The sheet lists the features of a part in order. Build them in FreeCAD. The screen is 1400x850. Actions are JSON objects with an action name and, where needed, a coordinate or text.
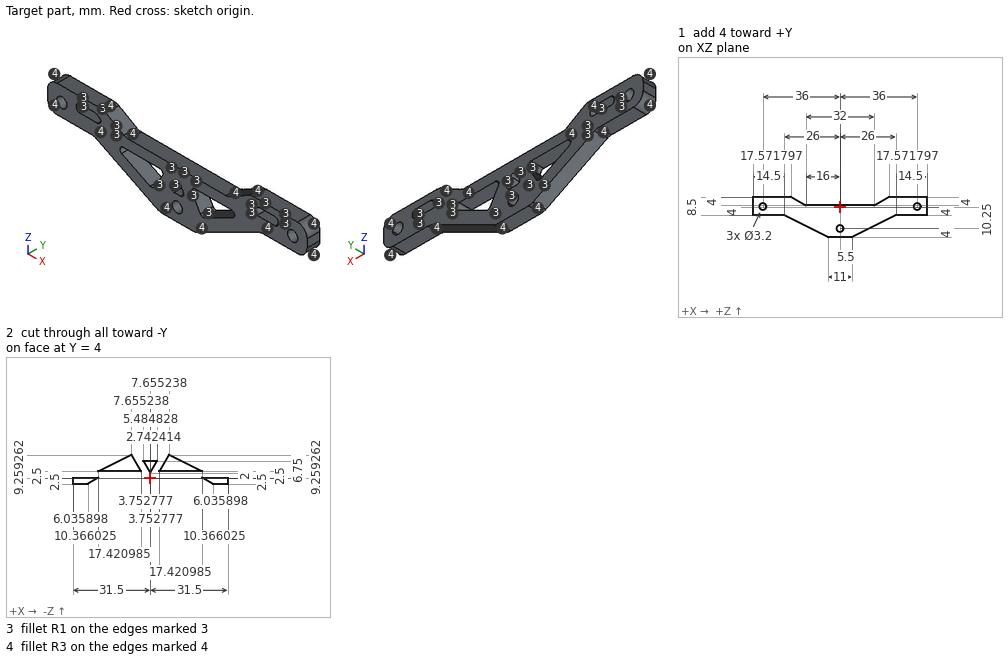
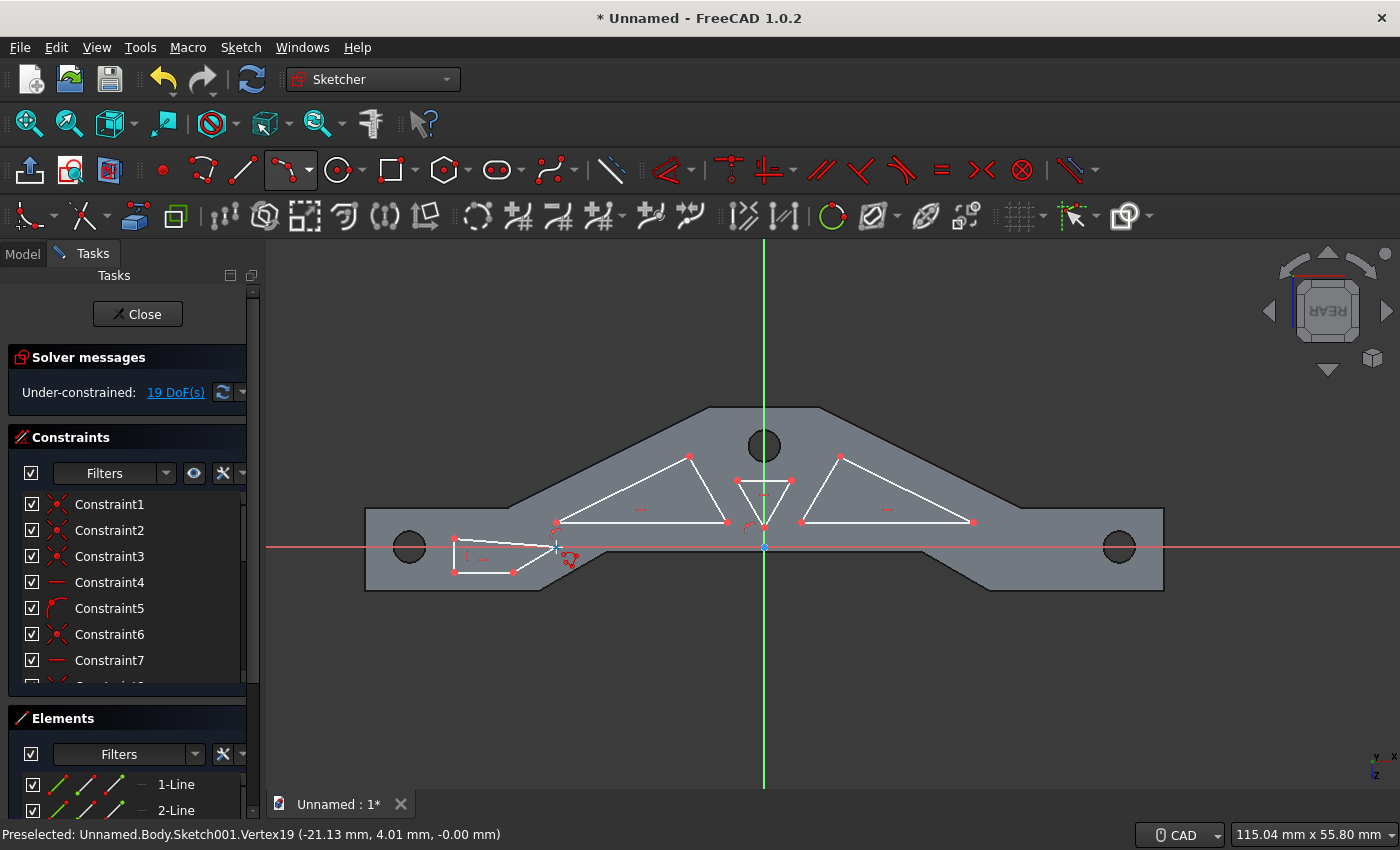
{"action": "left_click", "coordinate": [973, 547]}
{"action": "left_click", "coordinate": [1015, 572]}
{"action": "left_click", "coordinate": [1075, 572]}
{"action": "left_click", "coordinate": [1075, 538]}
{"action": "left_click", "coordinate": [973, 547]}
{"action": "key", "text": "Escape"}
{"action": "key", "text": "Escape"}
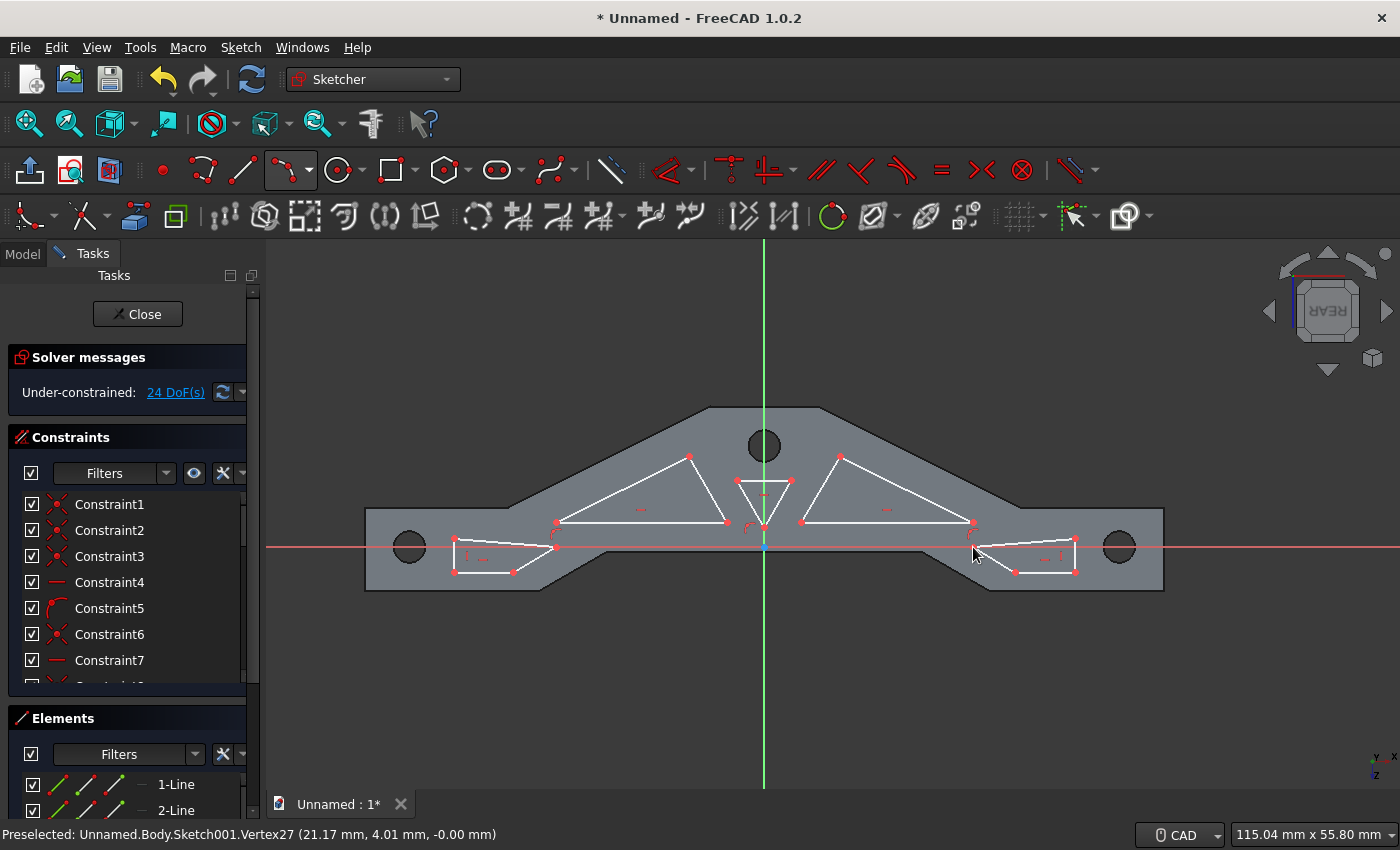
{"action": "left_click", "coordinate": [525, 545]}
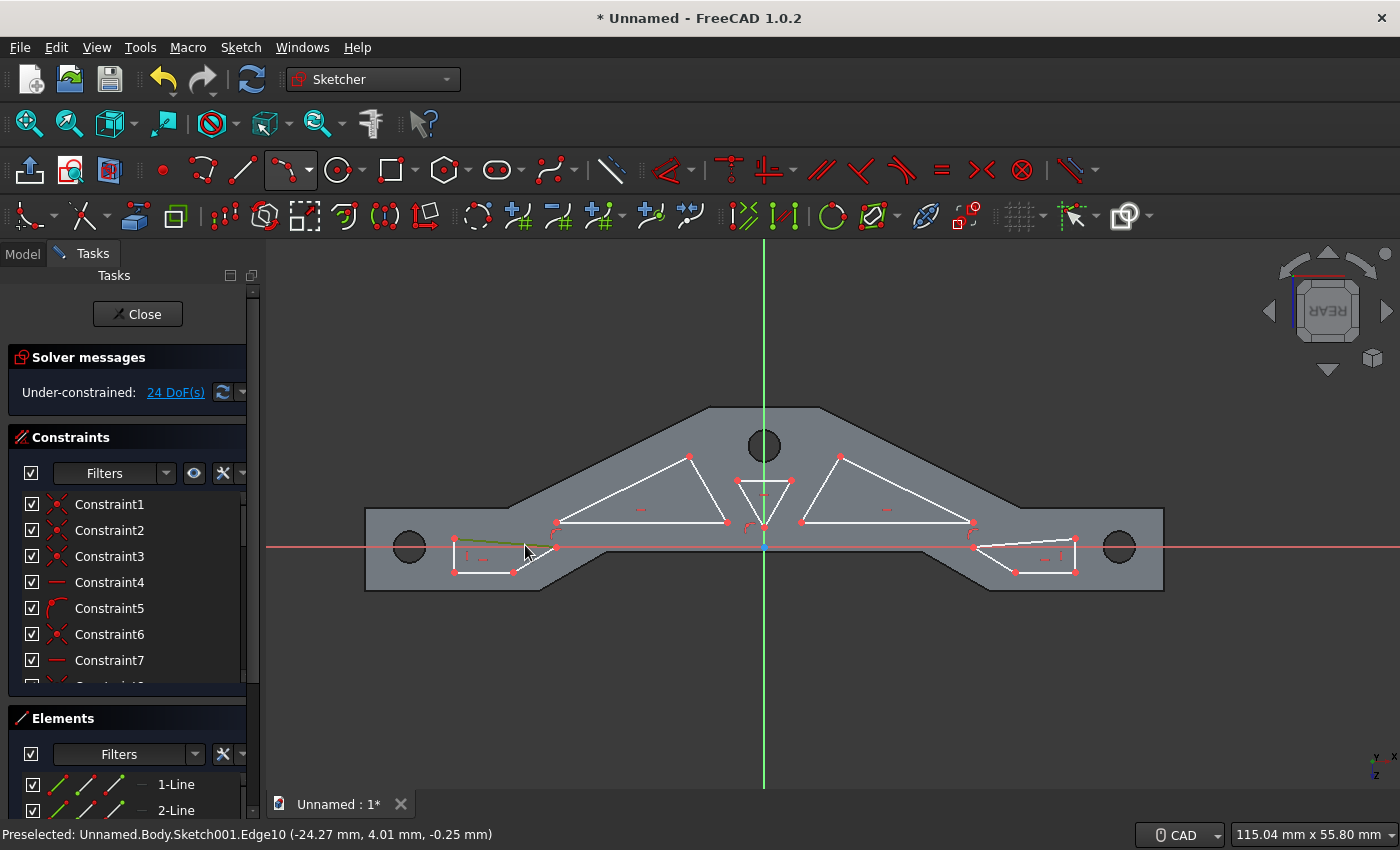
{"action": "key", "text": "h"}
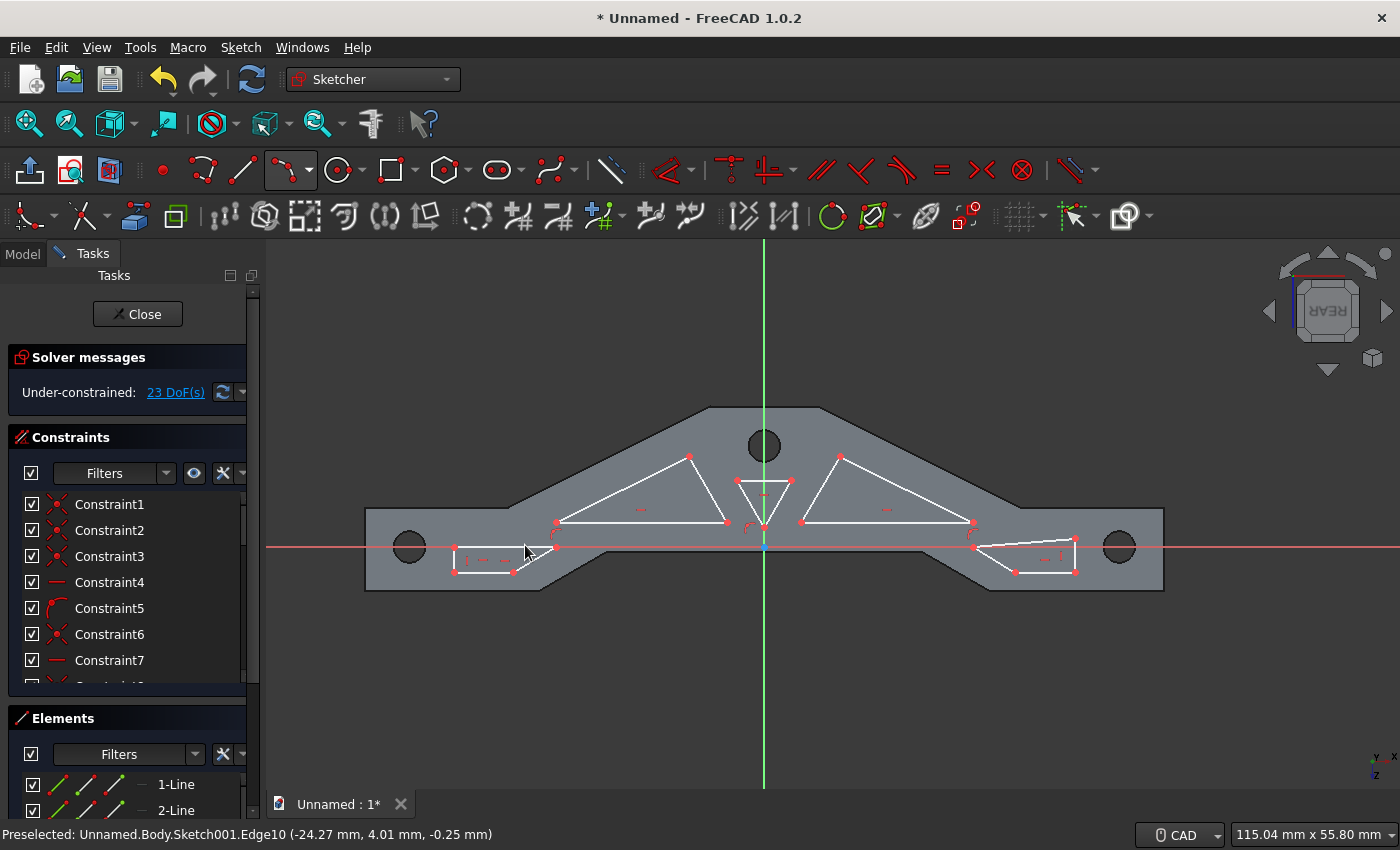
{"action": "left_click", "coordinate": [1004, 545]}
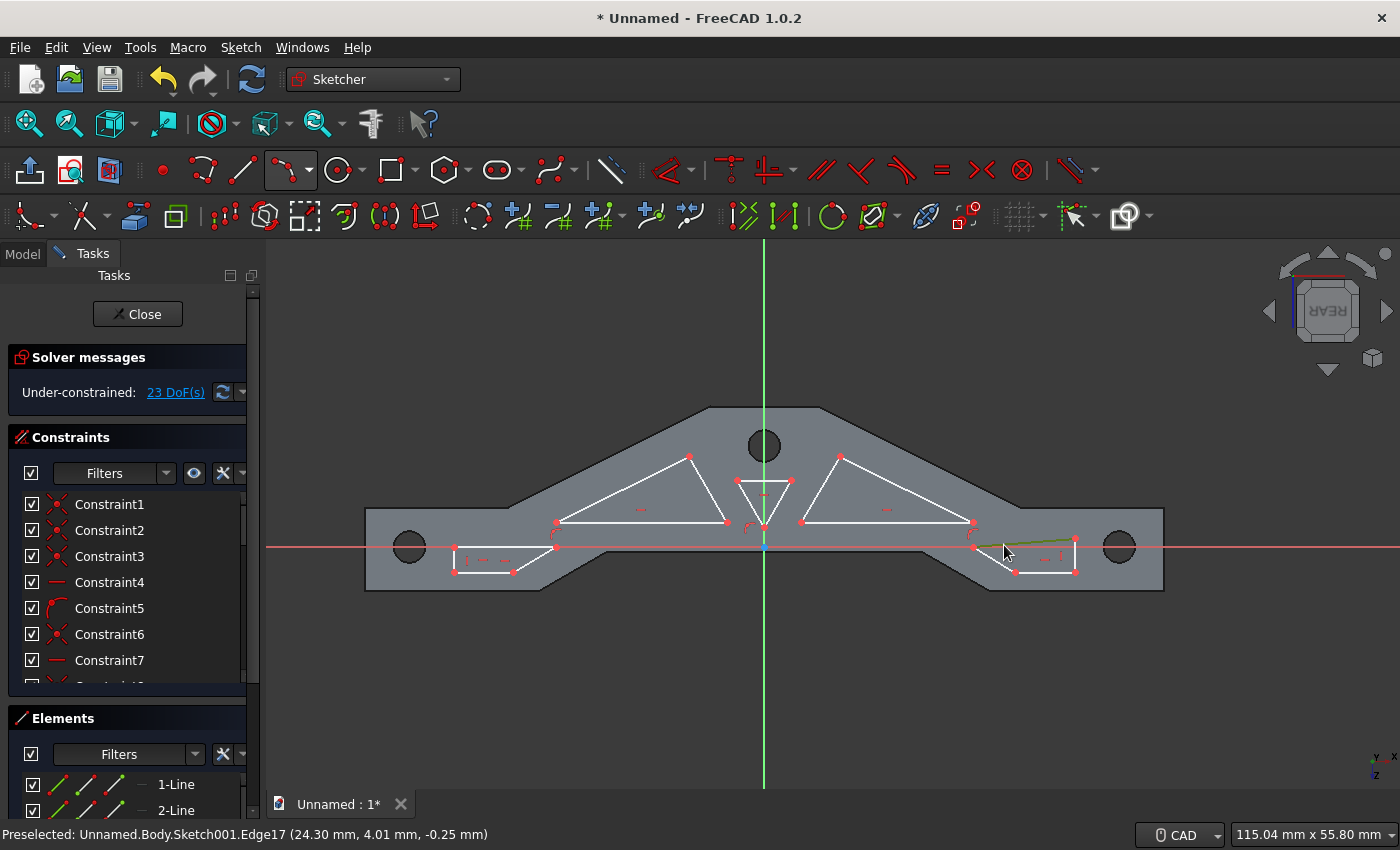
{"action": "left_click", "coordinate": [796, 170]}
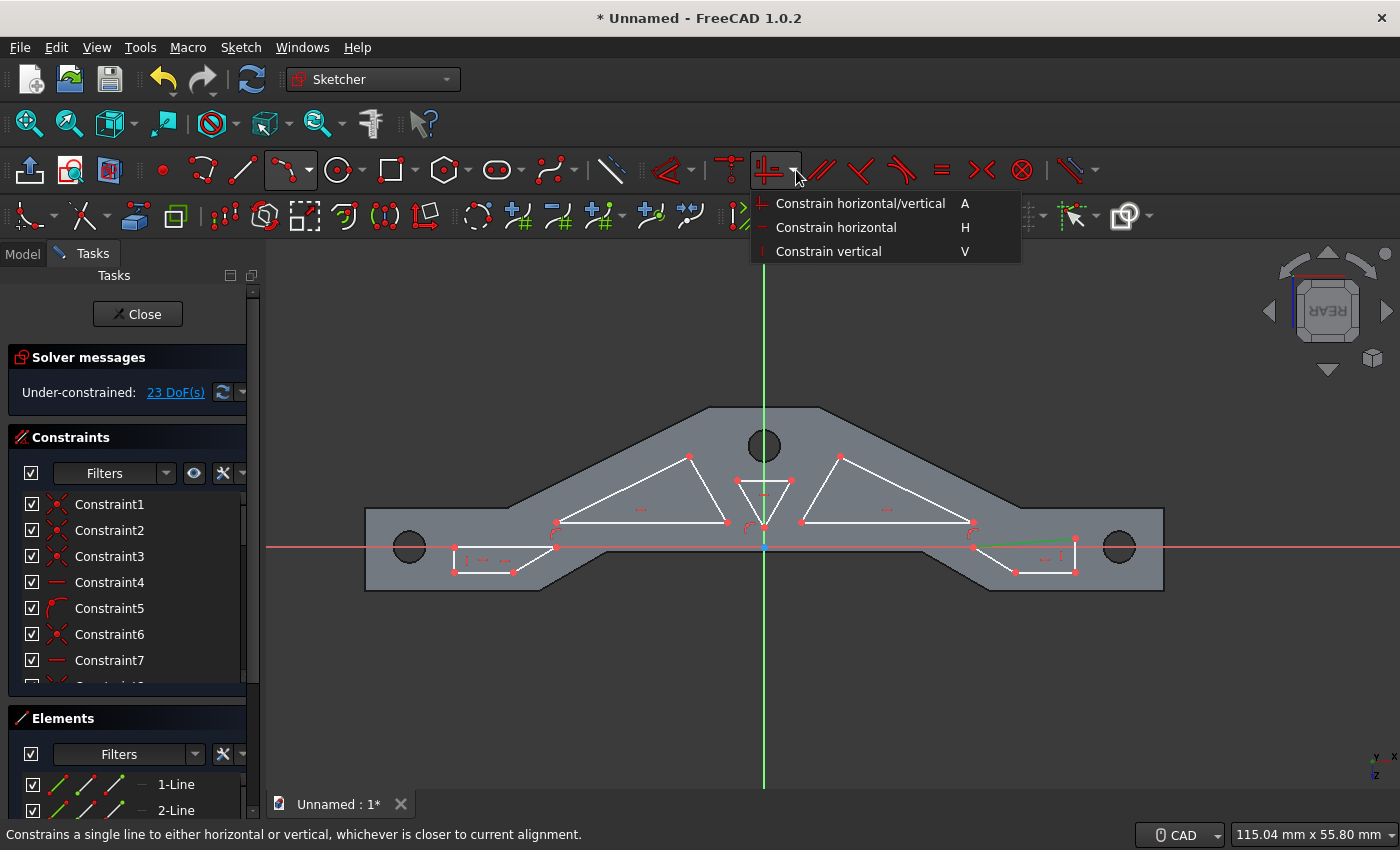
{"action": "left_click", "coordinate": [886, 227]}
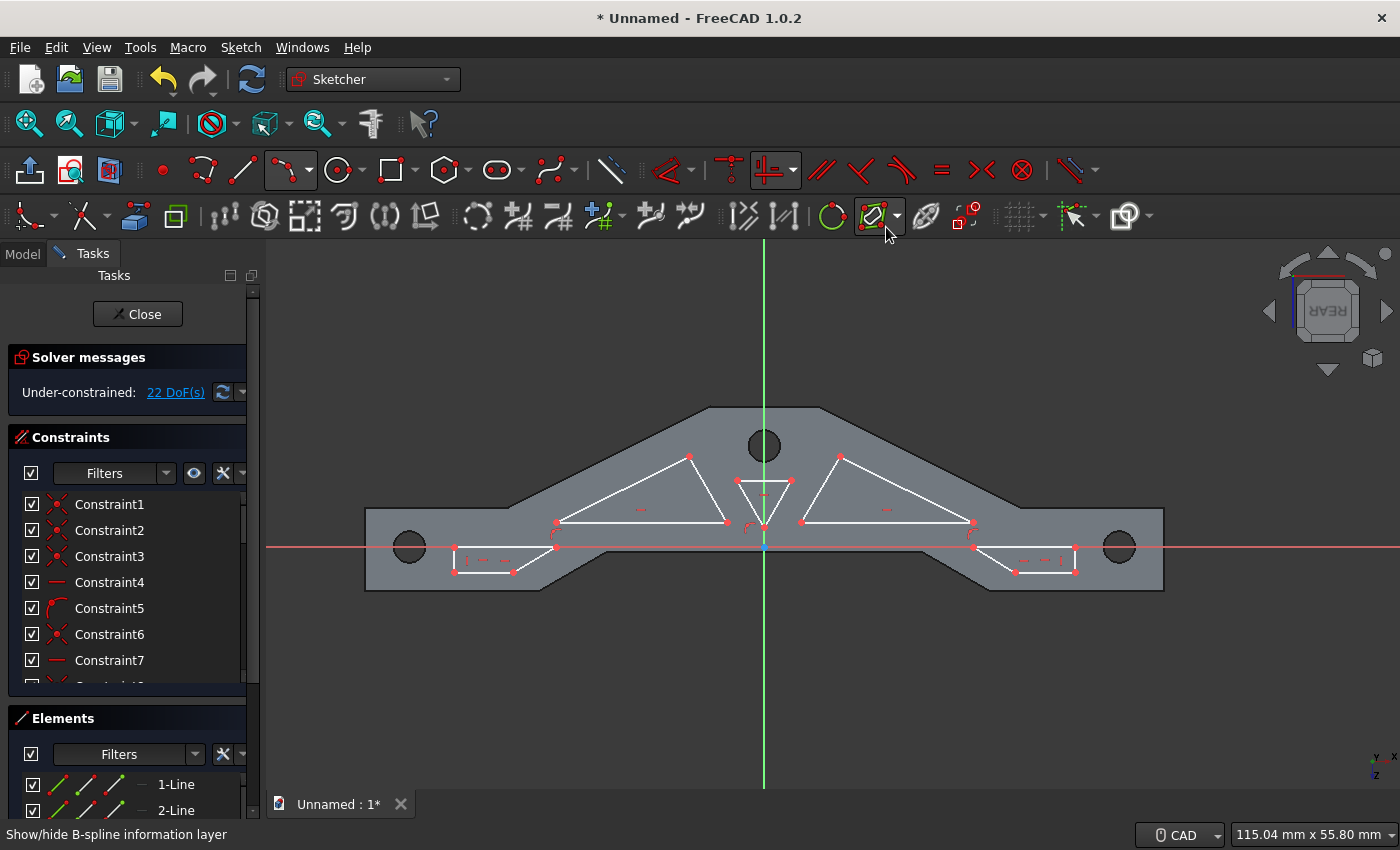
{"action": "left_click", "coordinate": [666, 170]}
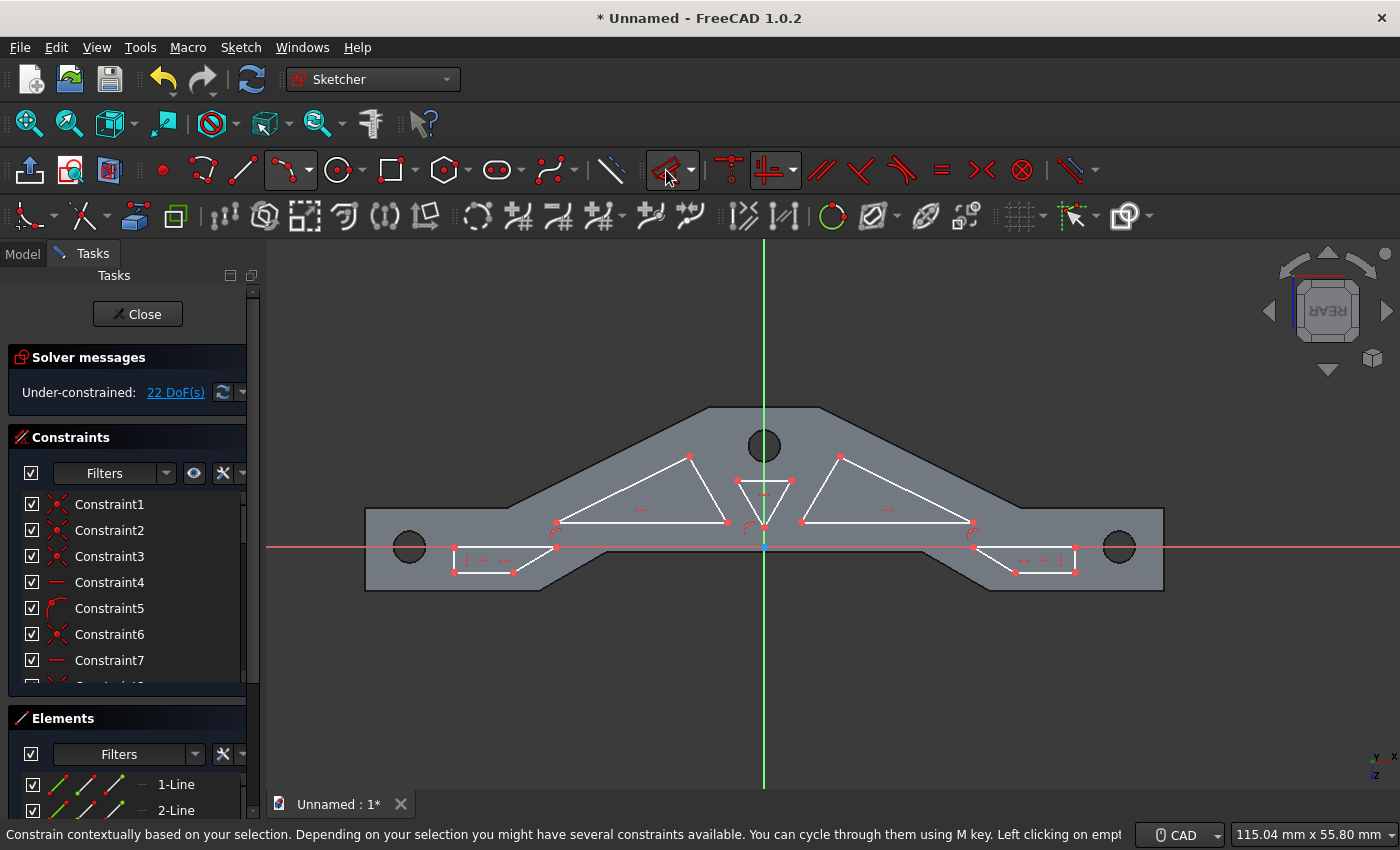
{"action": "scroll", "coordinate": [764, 528], "scroll_direction": "up", "scroll_amount": 4}